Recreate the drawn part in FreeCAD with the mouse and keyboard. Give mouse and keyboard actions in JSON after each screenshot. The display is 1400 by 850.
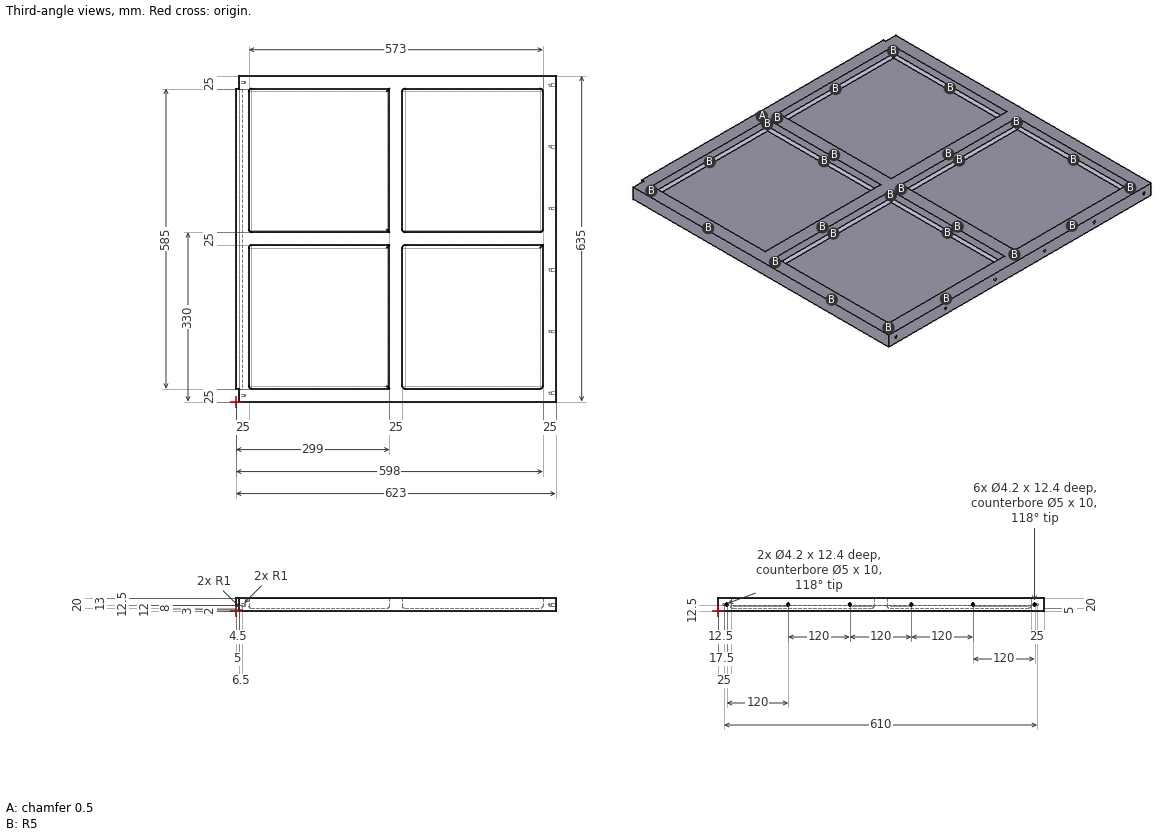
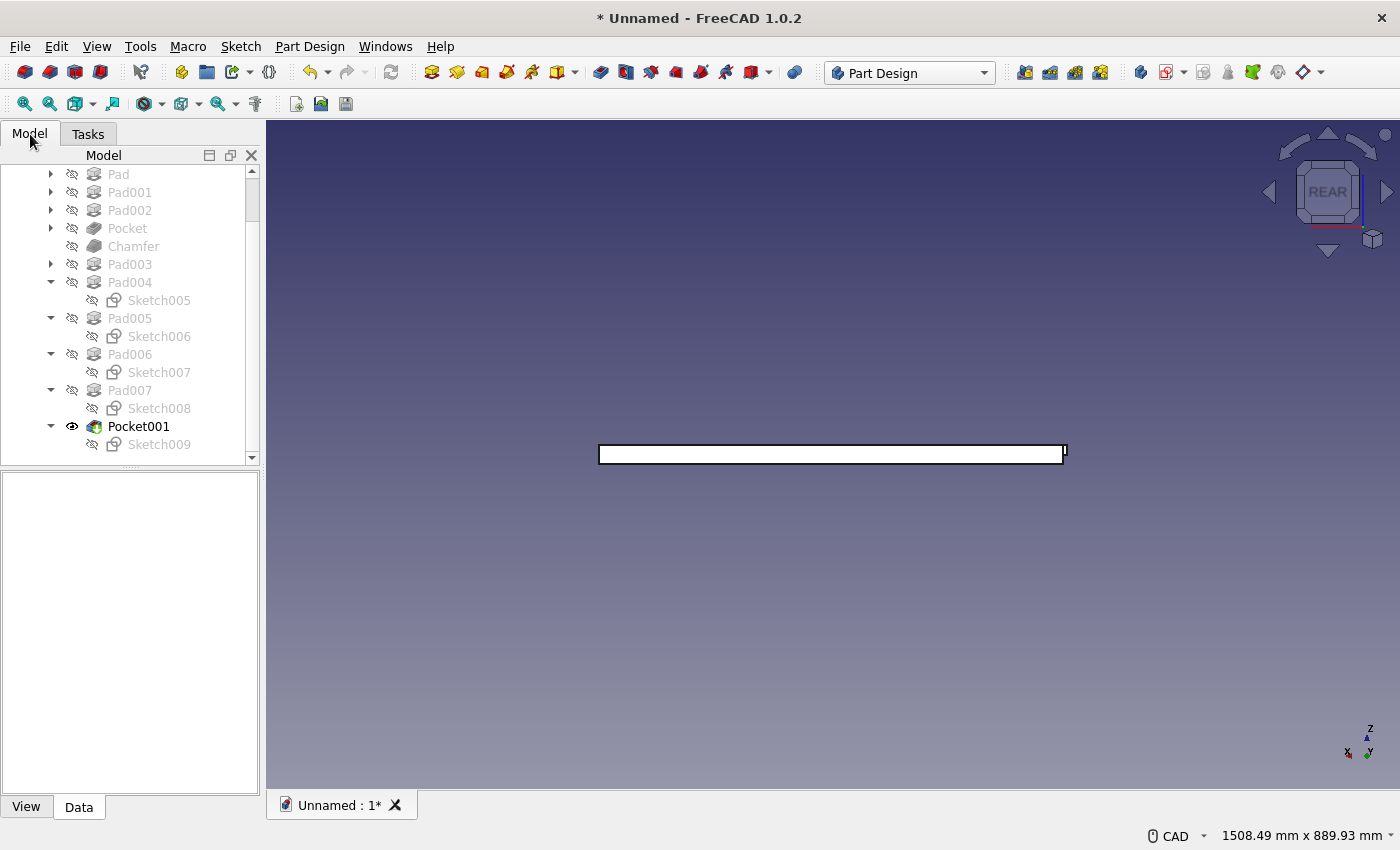
{"action": "scroll", "coordinate": [141, 314], "scroll_direction": "down", "scroll_amount": 3}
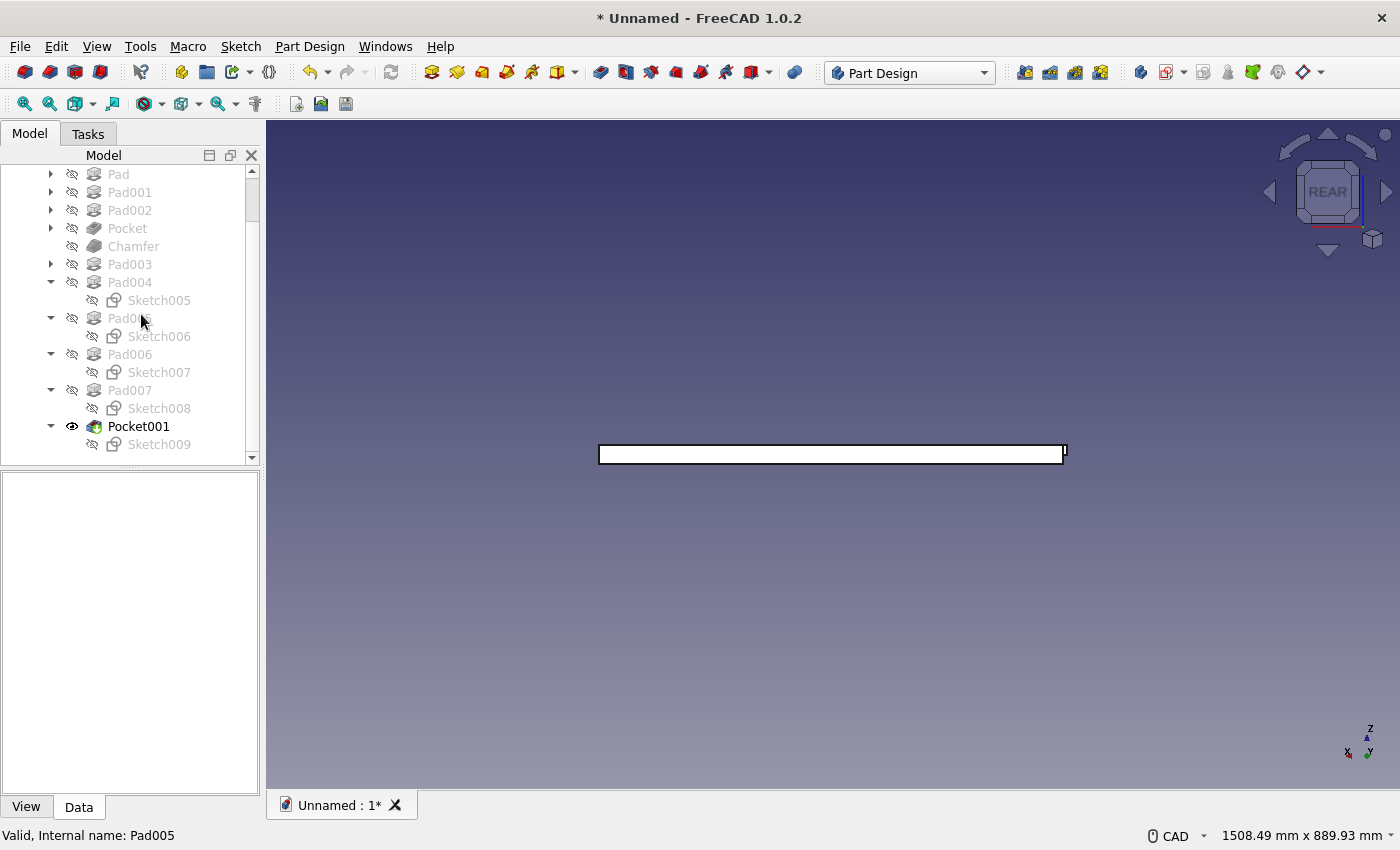
{"action": "scroll", "coordinate": [141, 314], "scroll_direction": "up", "scroll_amount": 15}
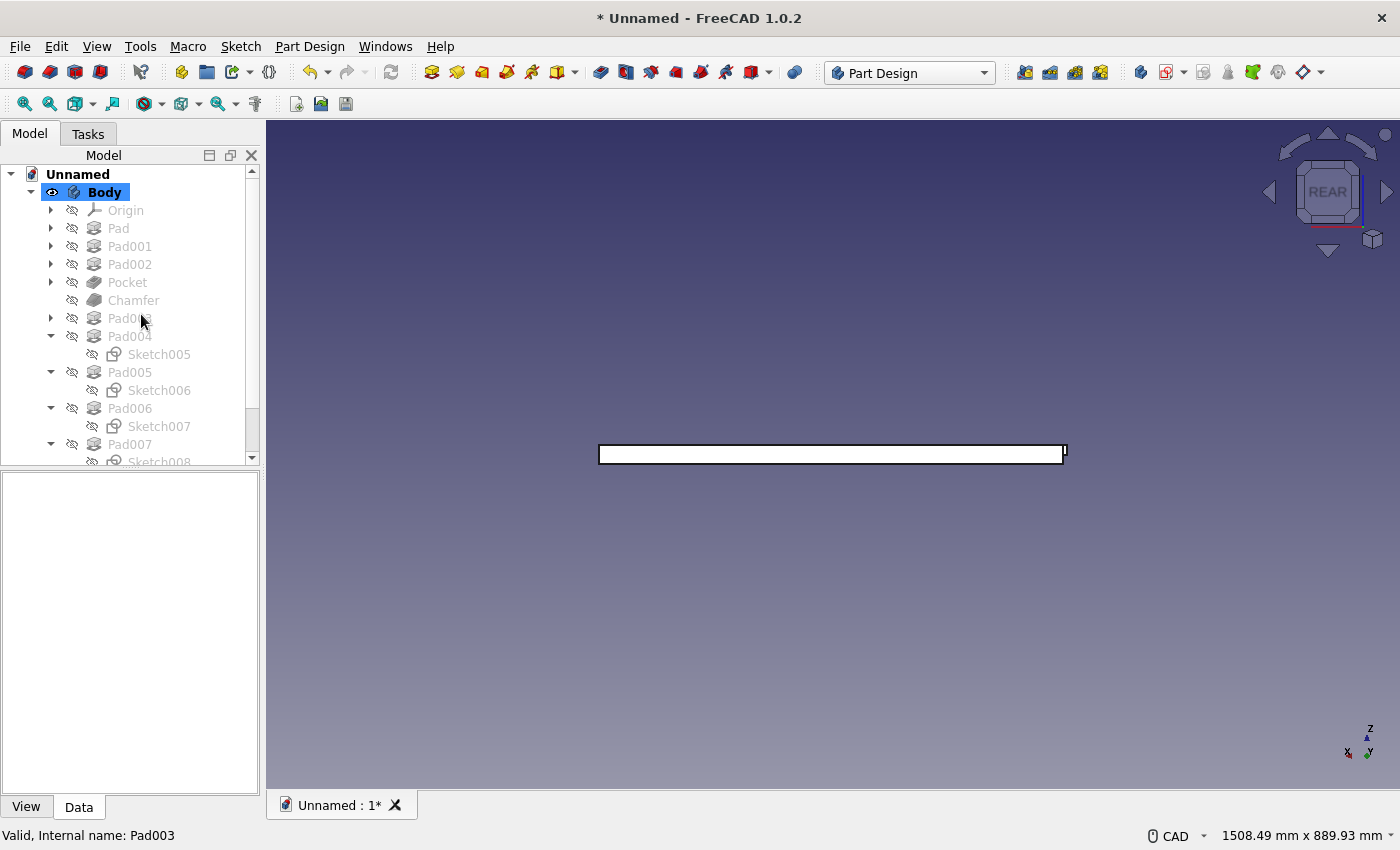
{"action": "left_click", "coordinate": [51, 210]}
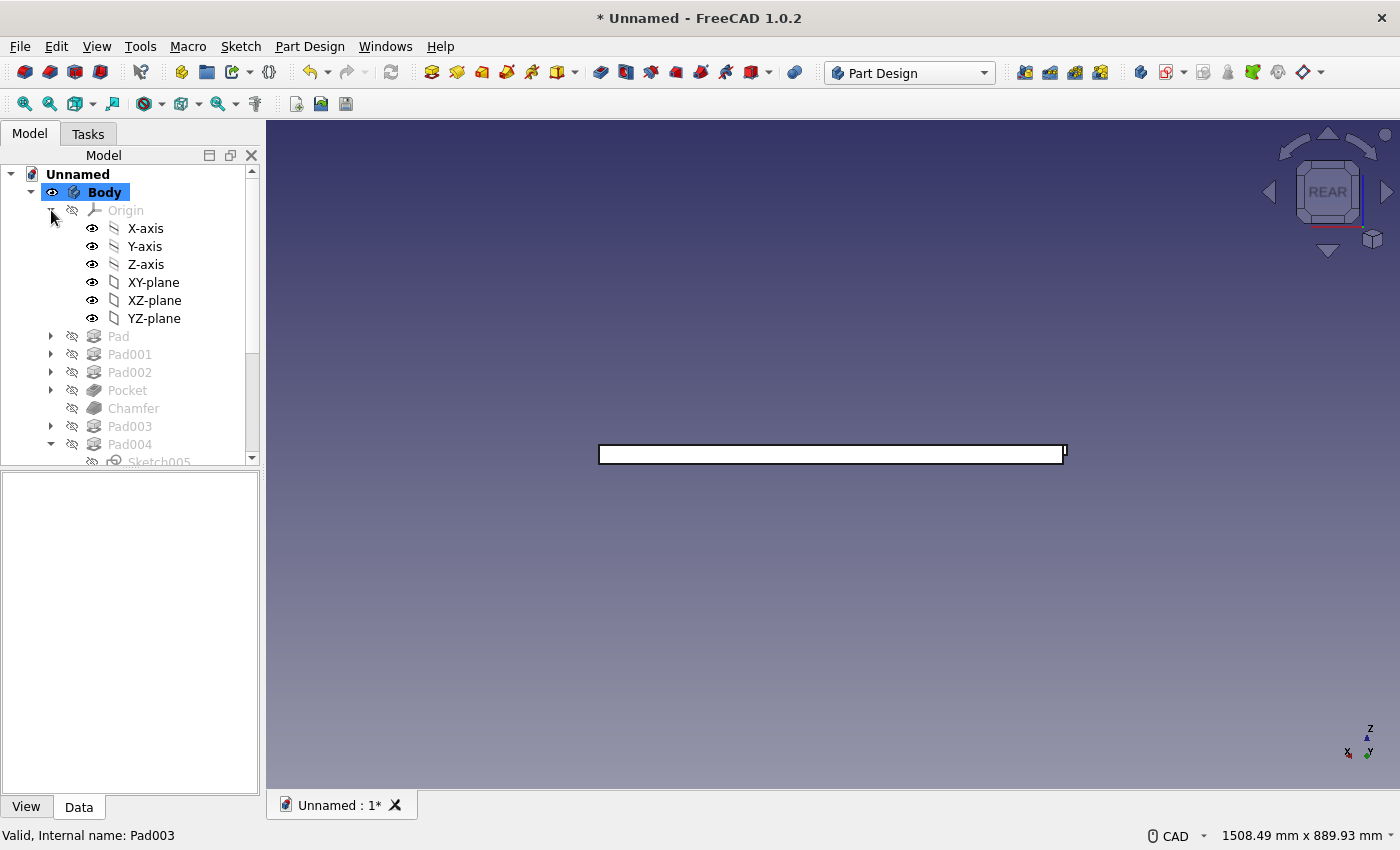
{"action": "left_click", "coordinate": [137, 300]}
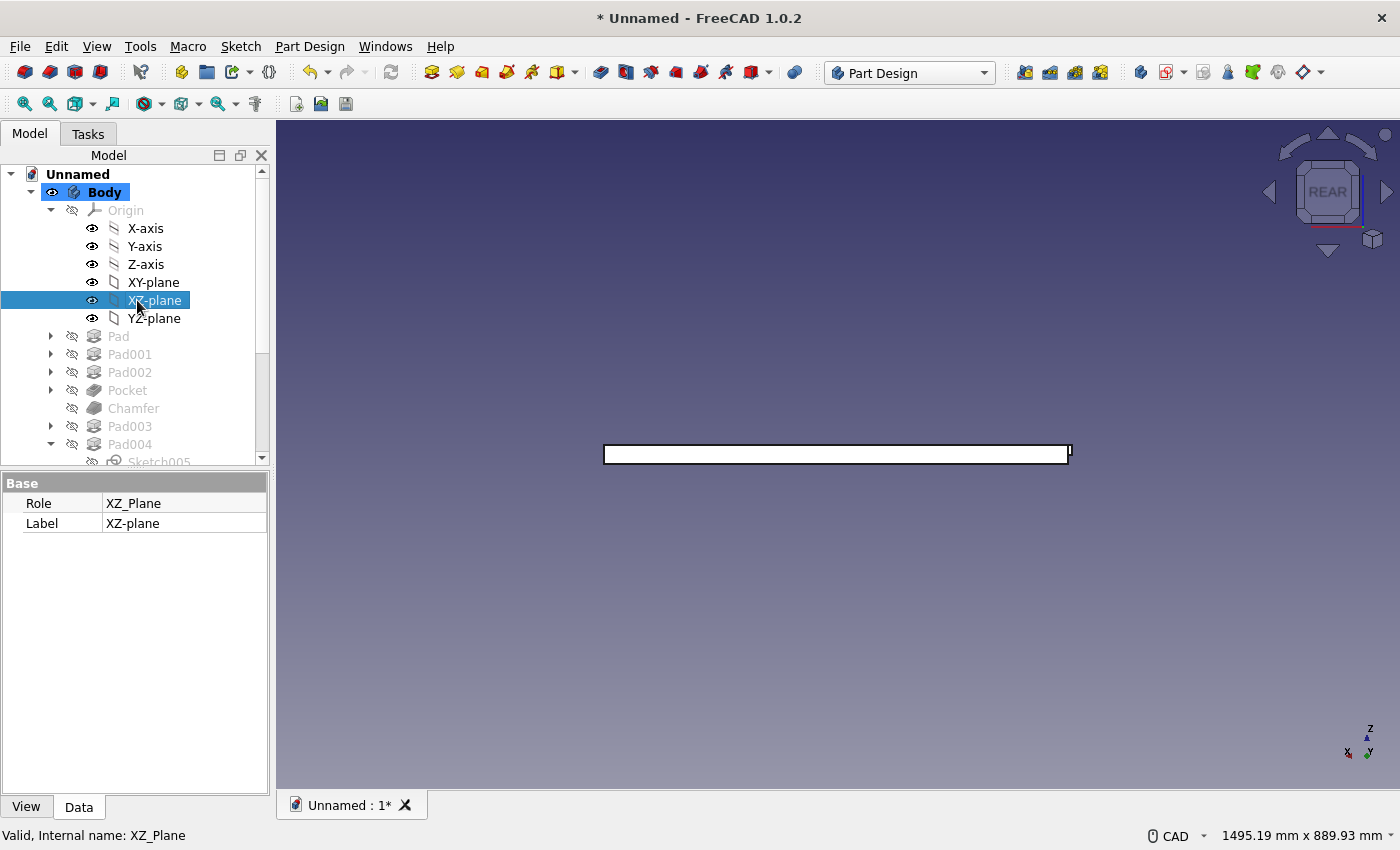
{"action": "left_click", "coordinate": [1302, 72]}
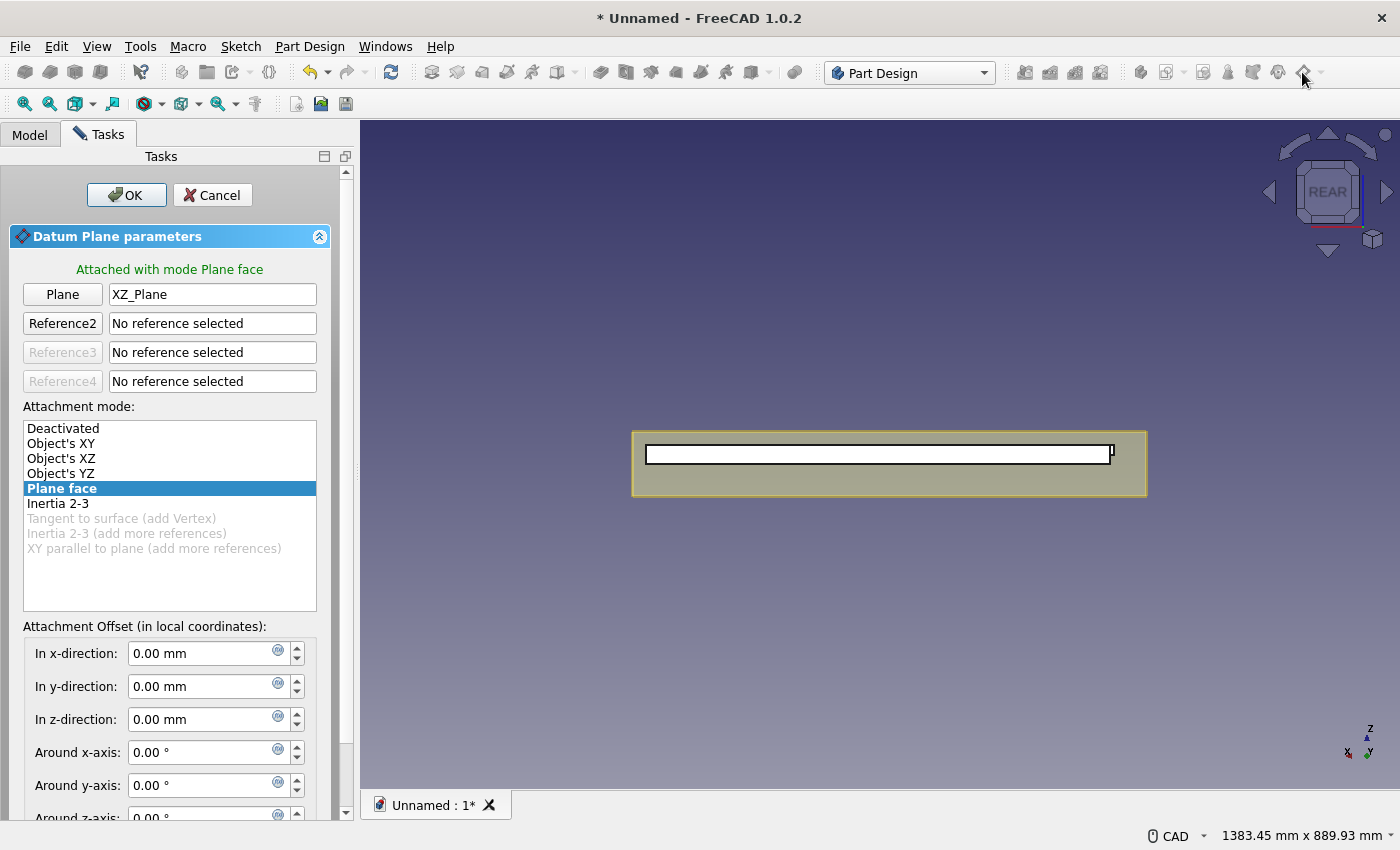
{"action": "triple_click", "coordinate": [210, 720]}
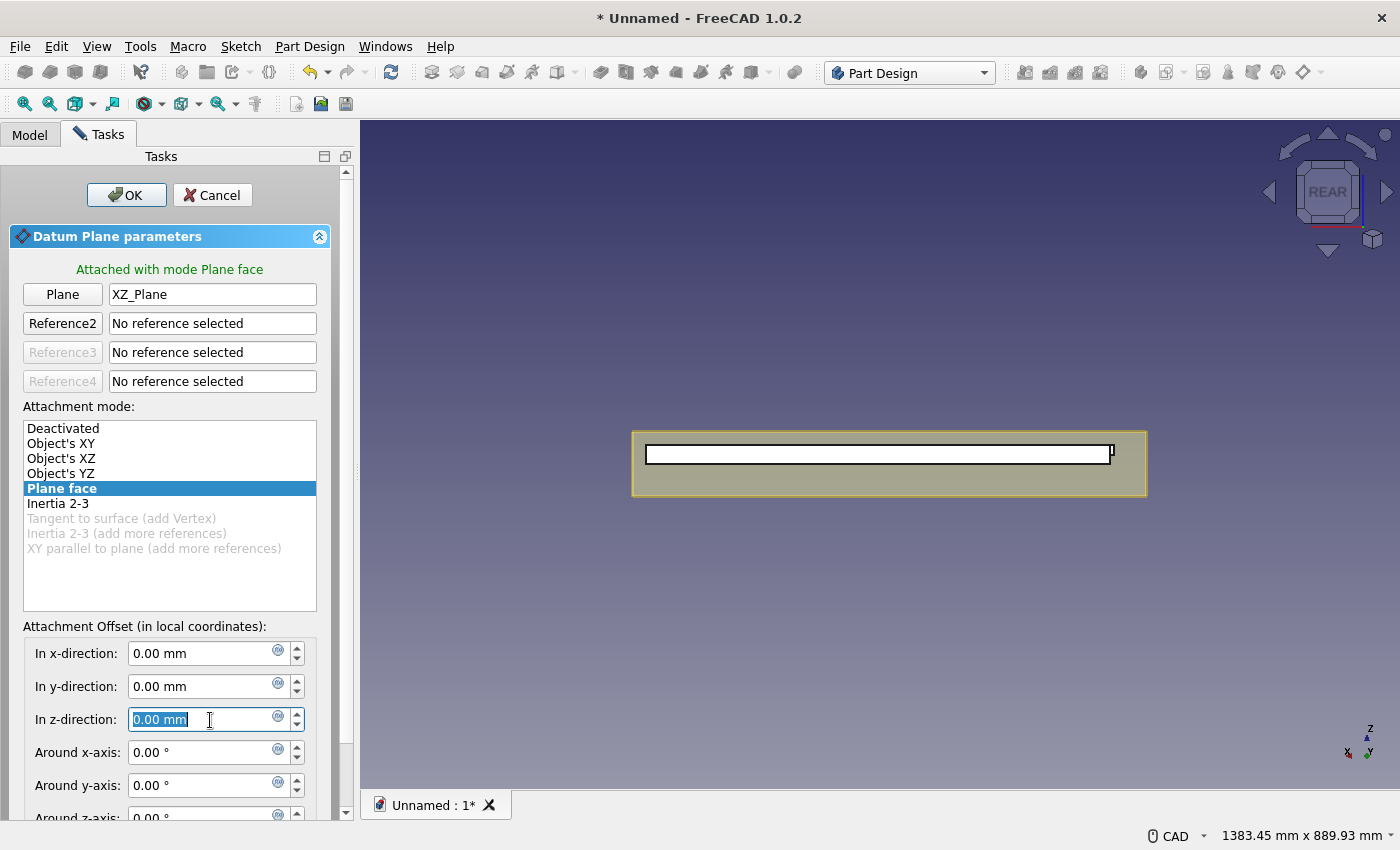
{"action": "type", "text": "-25"}
{"action": "key", "text": "Tab"}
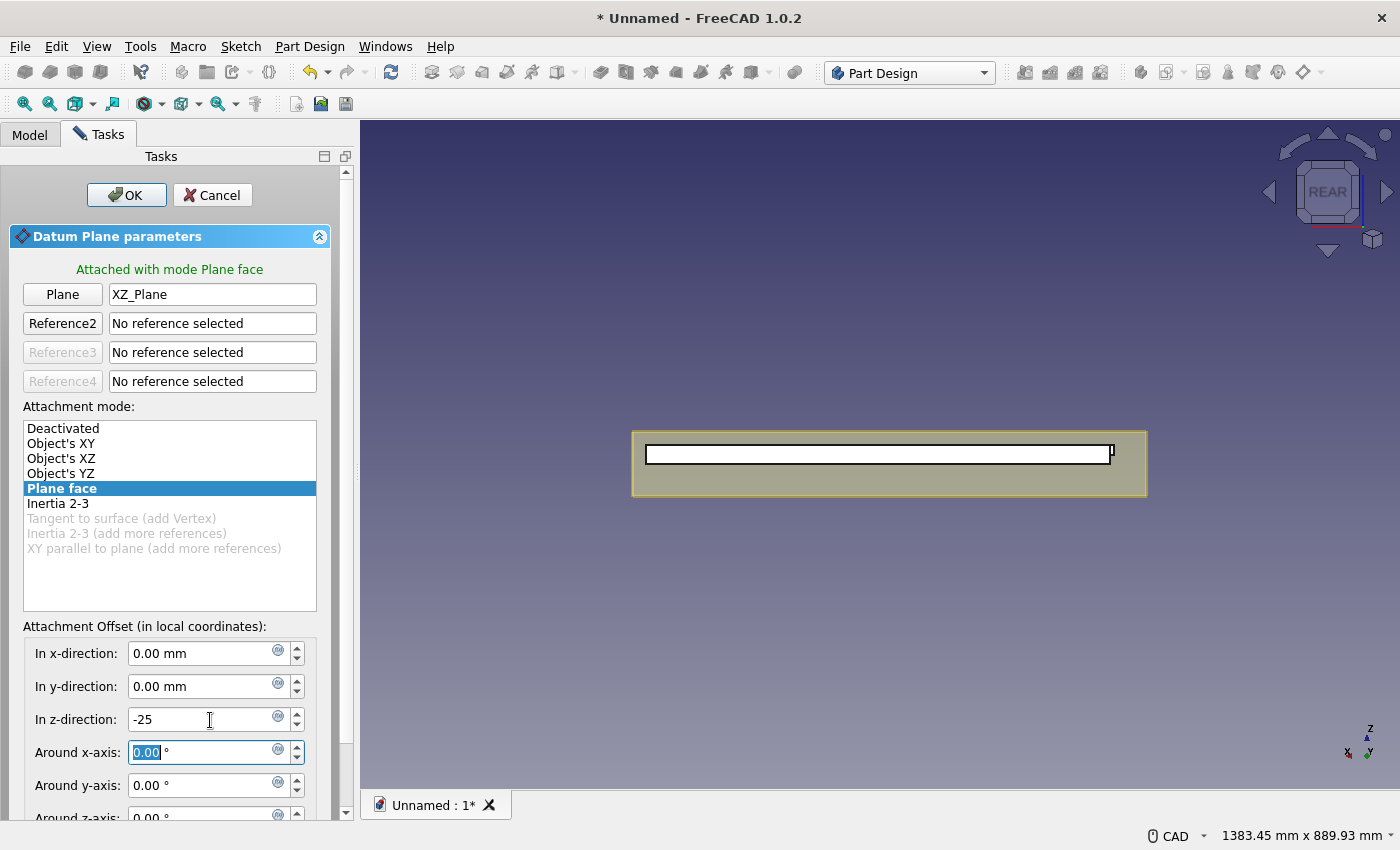
{"action": "left_click", "coordinate": [127, 195]}